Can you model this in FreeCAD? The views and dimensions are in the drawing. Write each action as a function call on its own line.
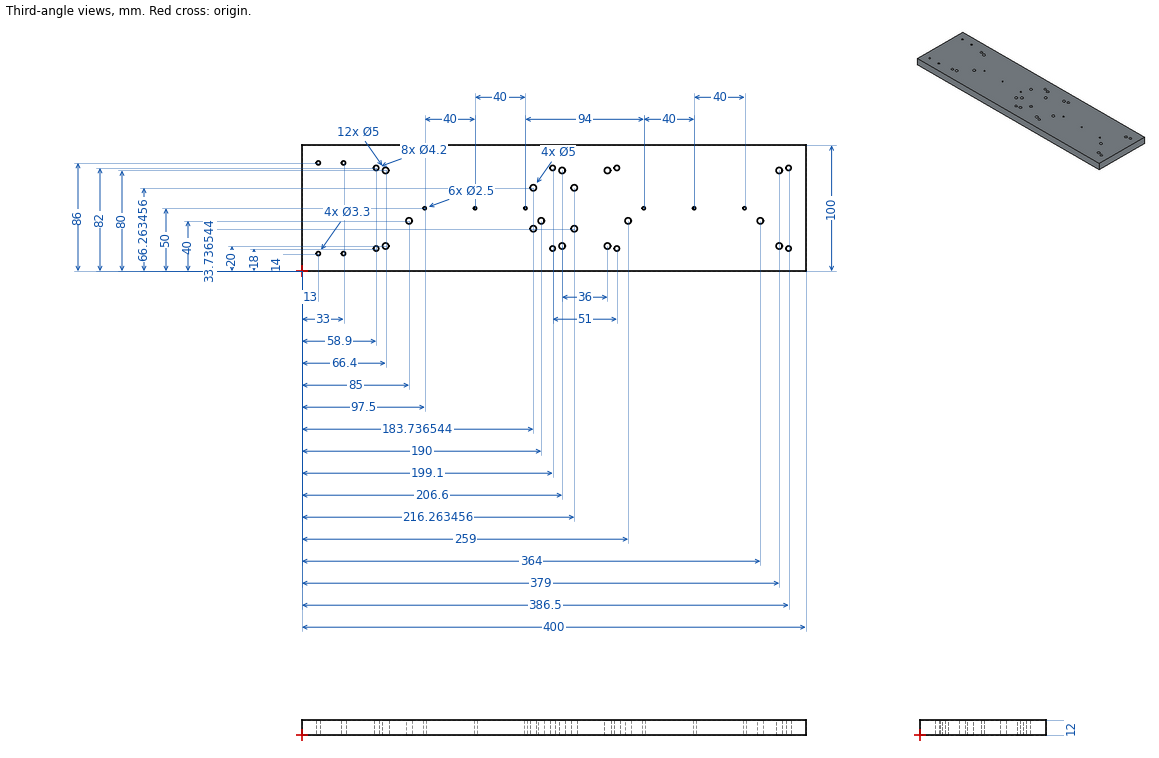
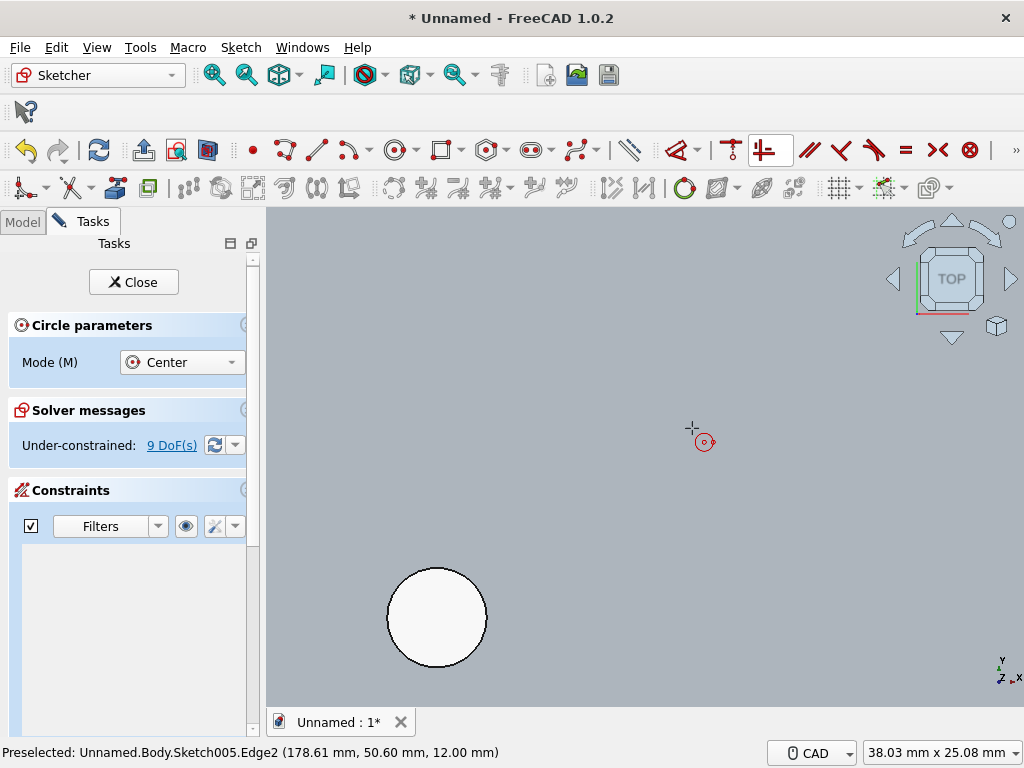
scroll(692, 428, down, 14)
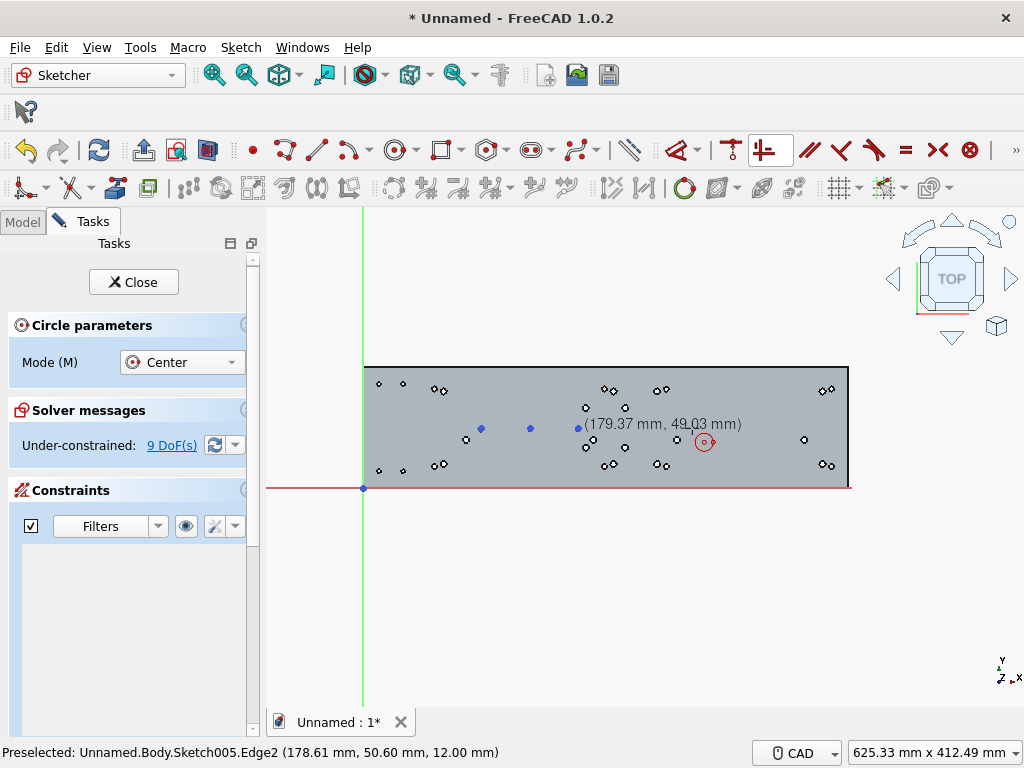
click(692, 428)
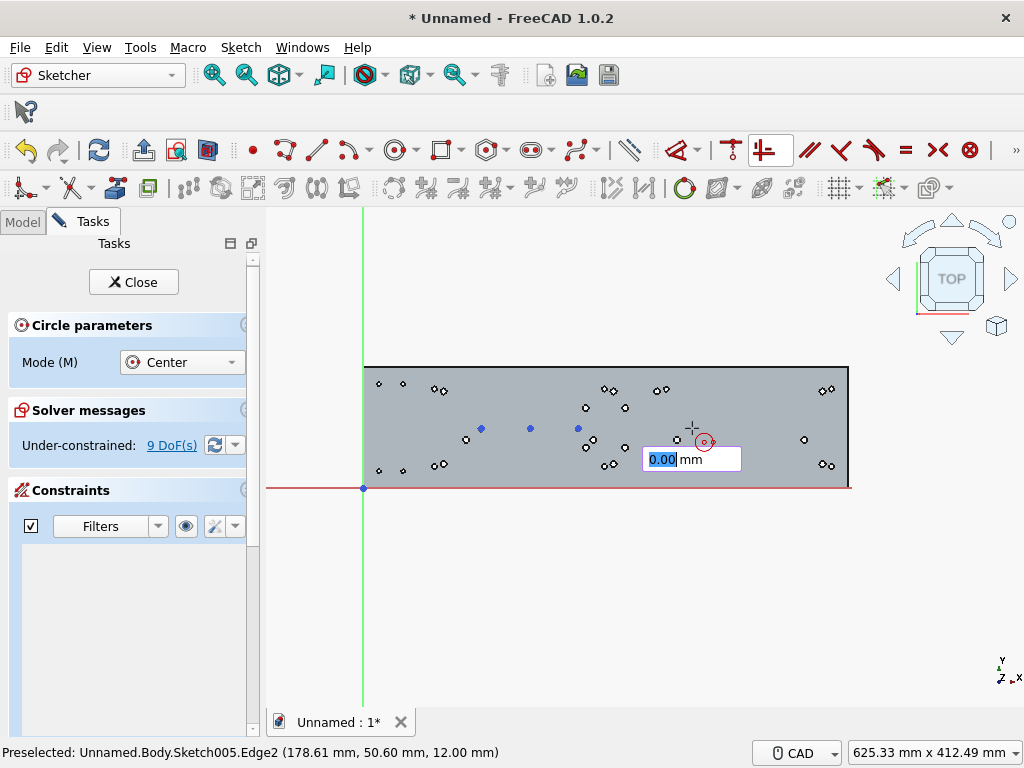
scroll(693, 427, up, 12)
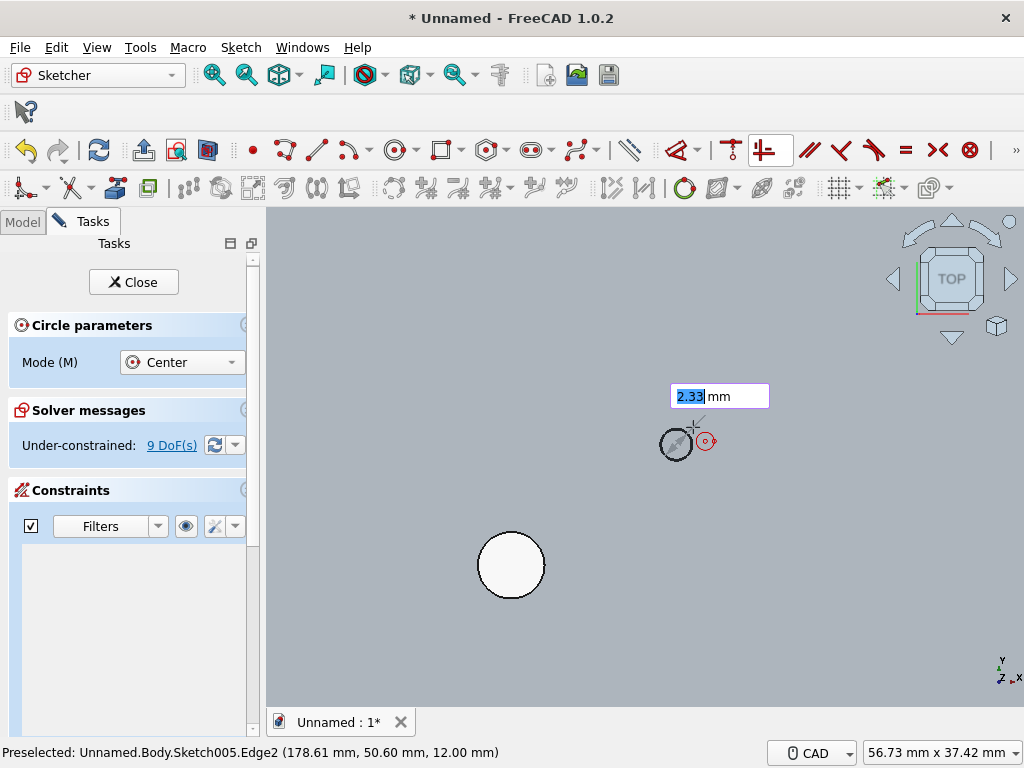
click(690, 420)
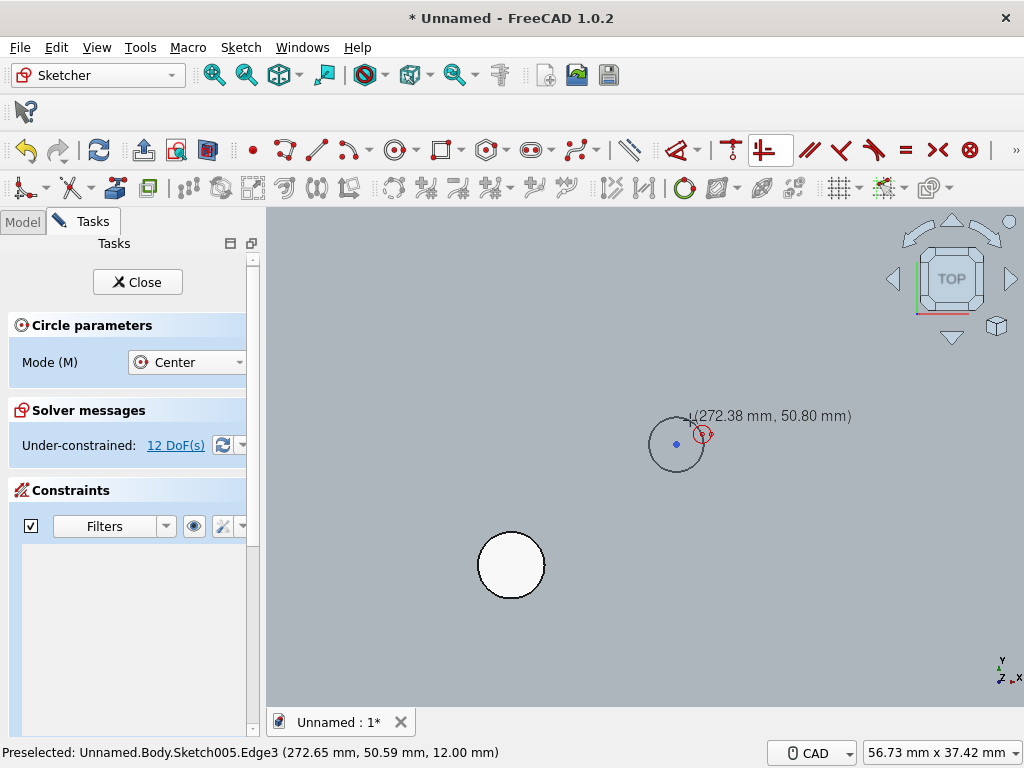
scroll(693, 427, down, 12)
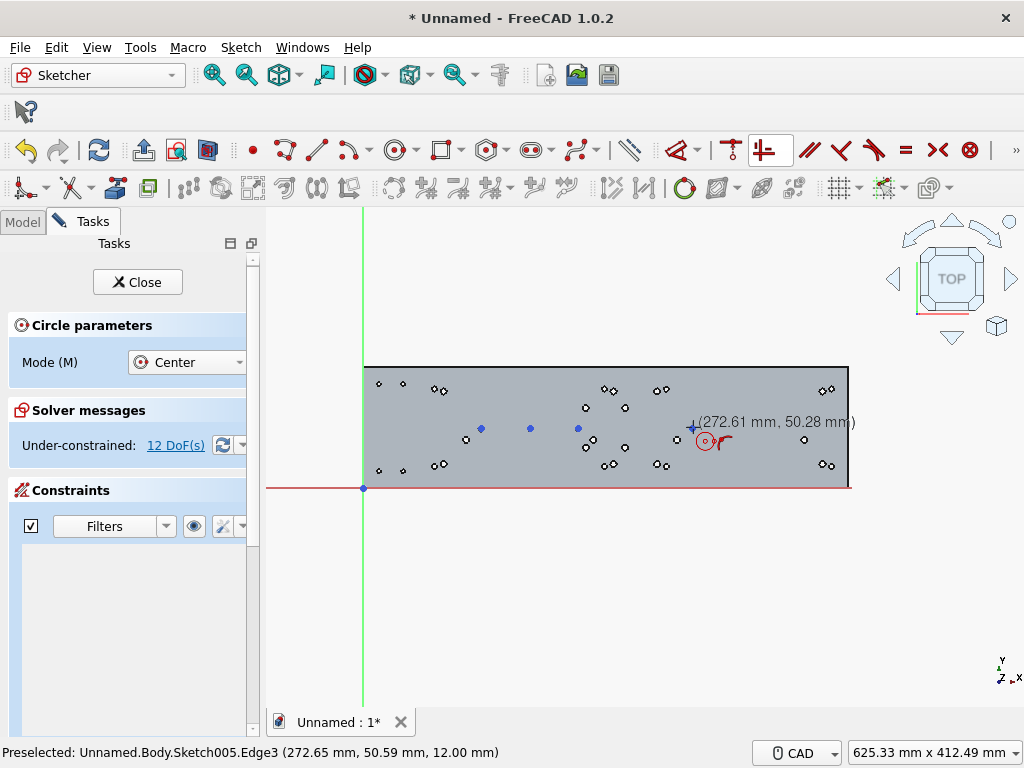
scroll(741, 428, up, 14)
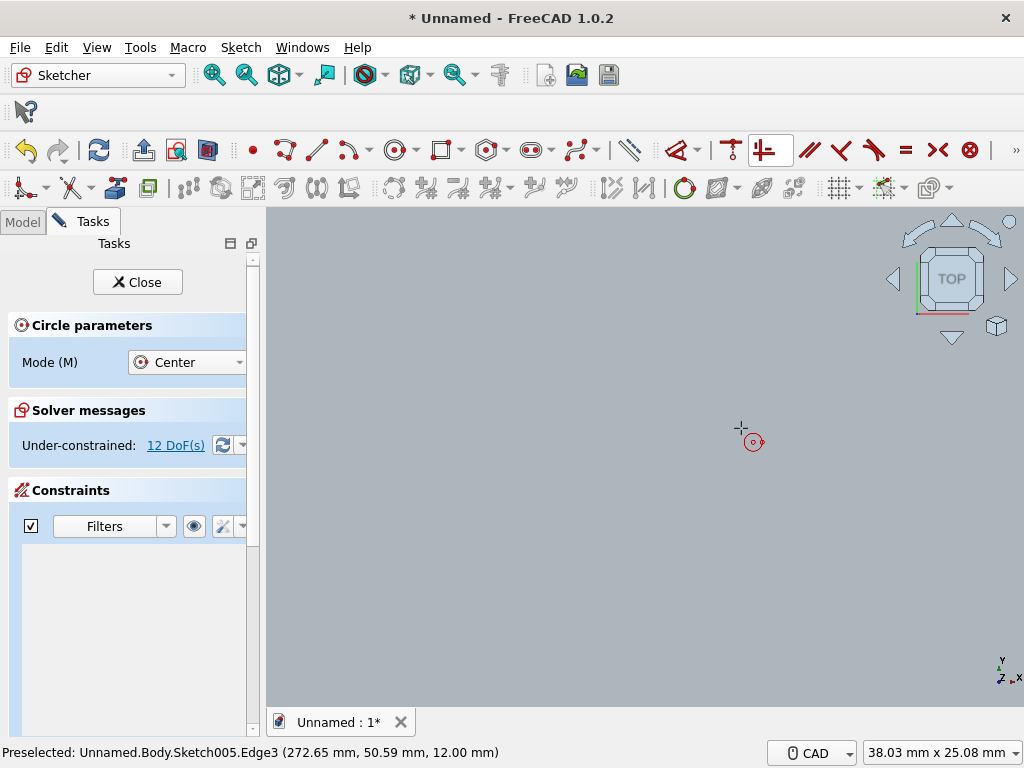
scroll(741, 428, down, 14)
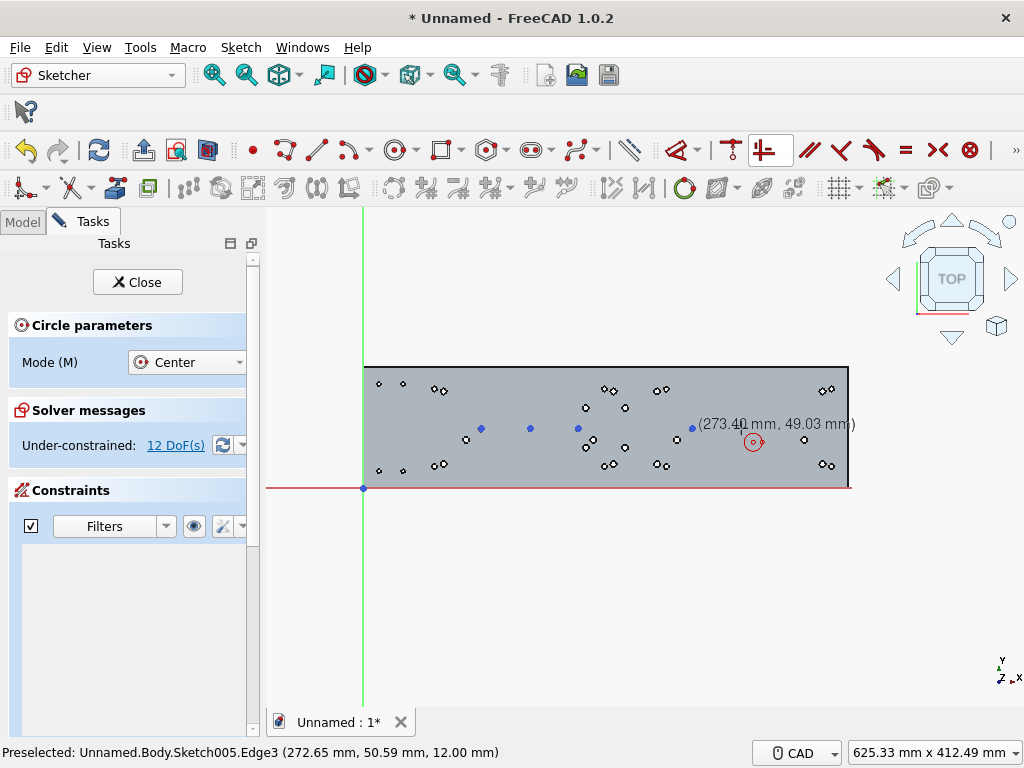
click(741, 428)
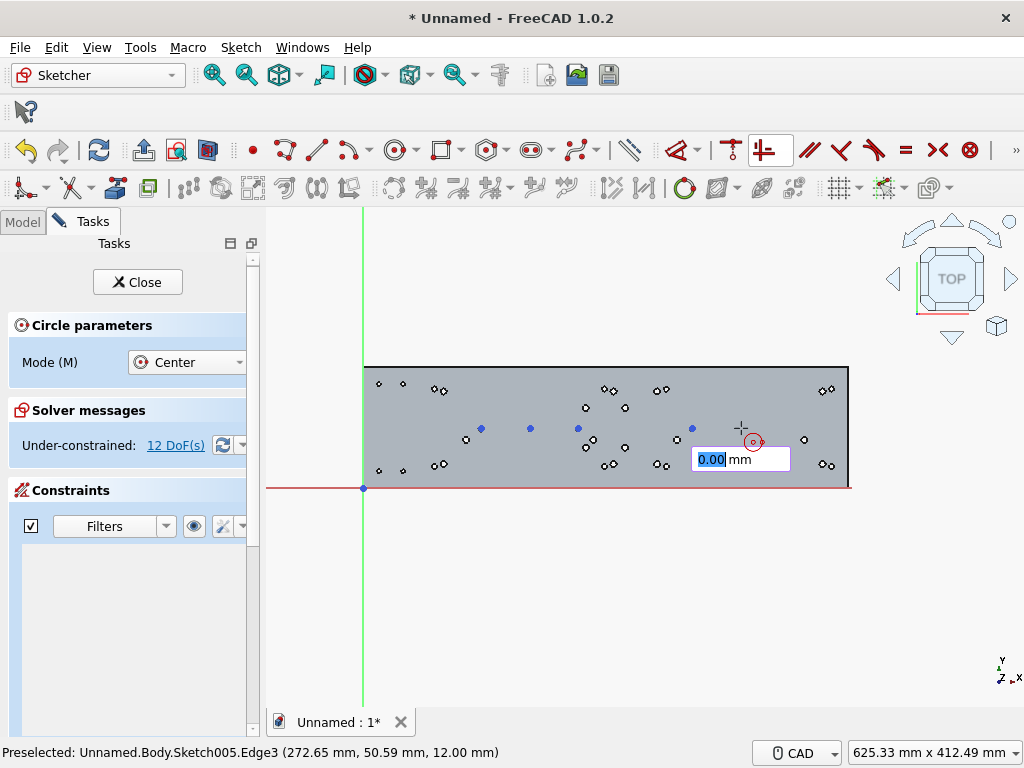
scroll(742, 427, up, 12)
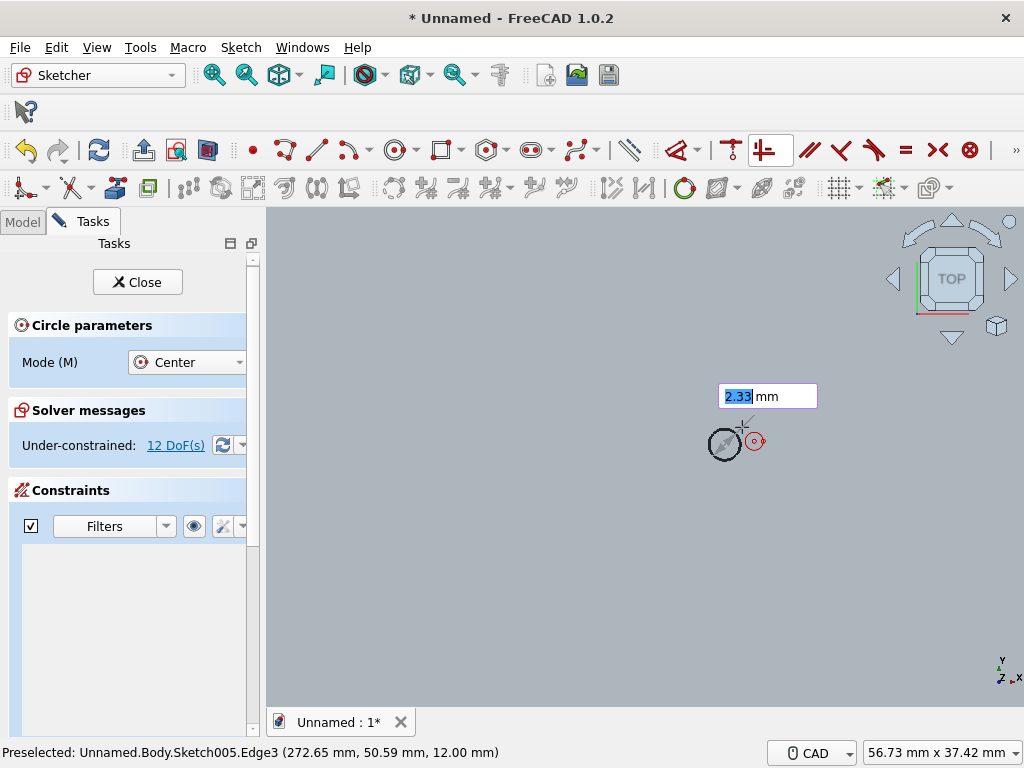
click(733, 420)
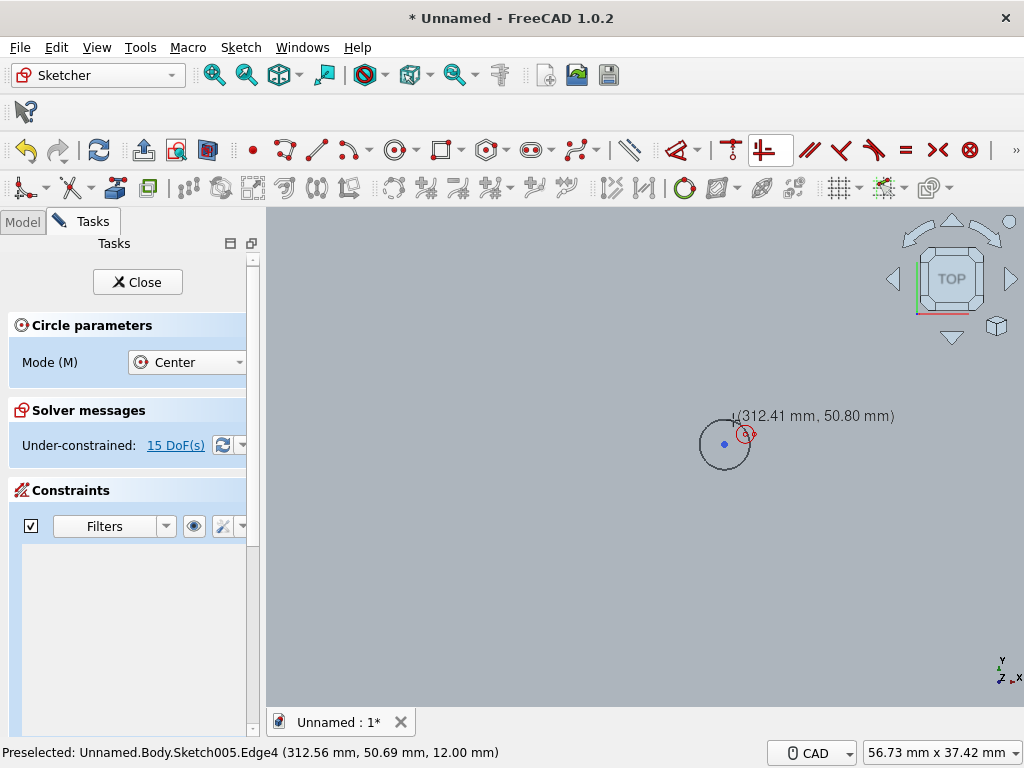
scroll(742, 427, down, 12)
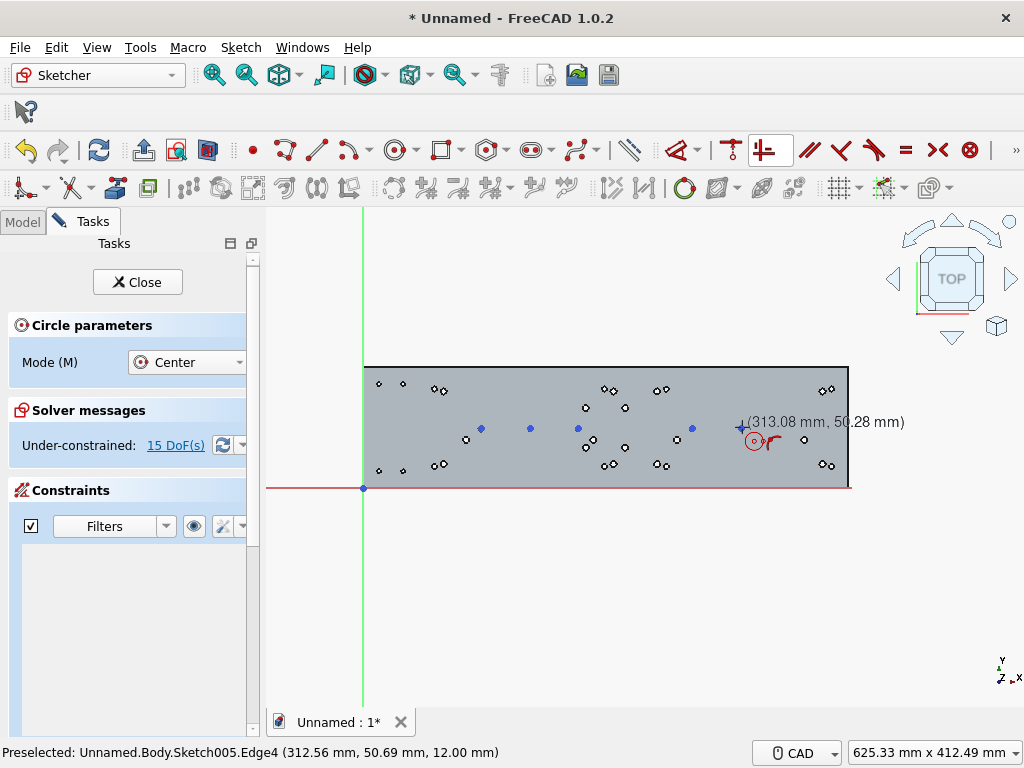
scroll(789, 428, up, 14)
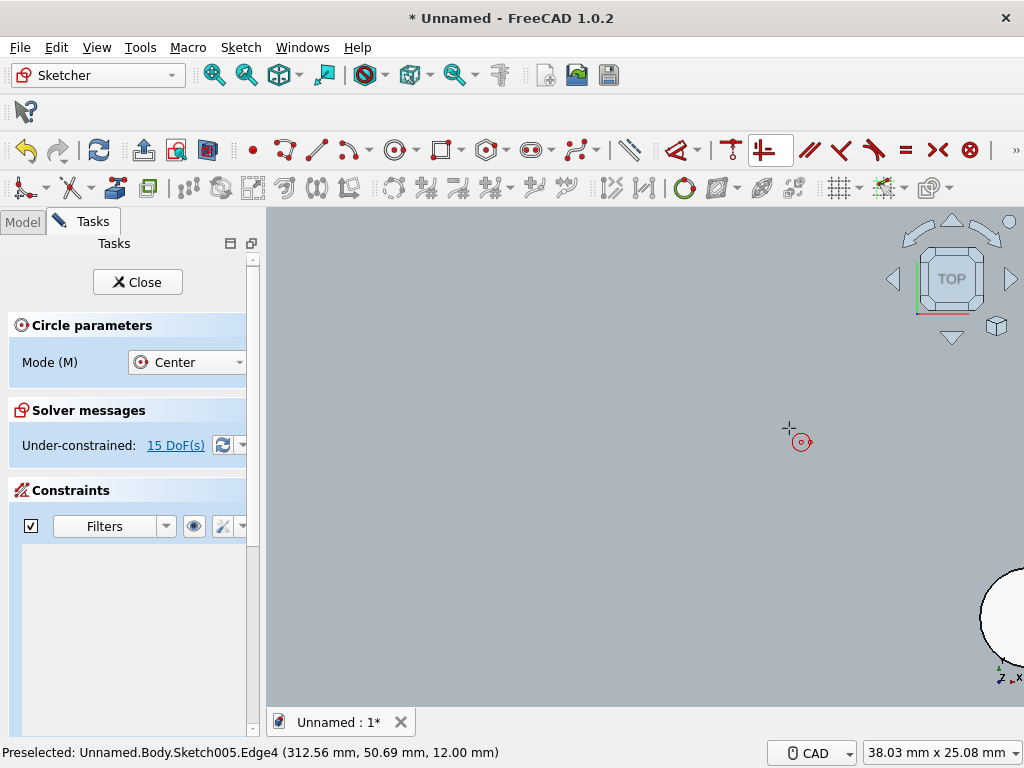
scroll(789, 428, down, 14)